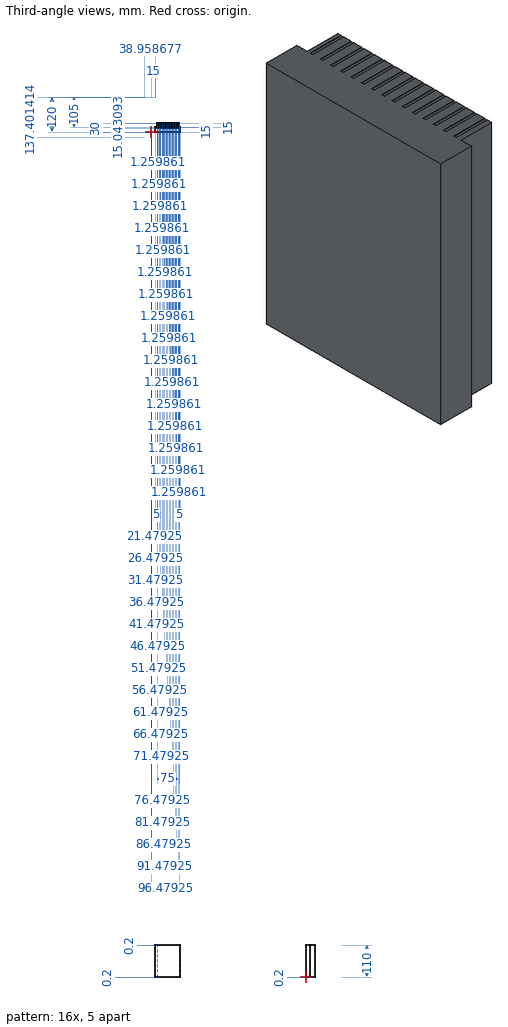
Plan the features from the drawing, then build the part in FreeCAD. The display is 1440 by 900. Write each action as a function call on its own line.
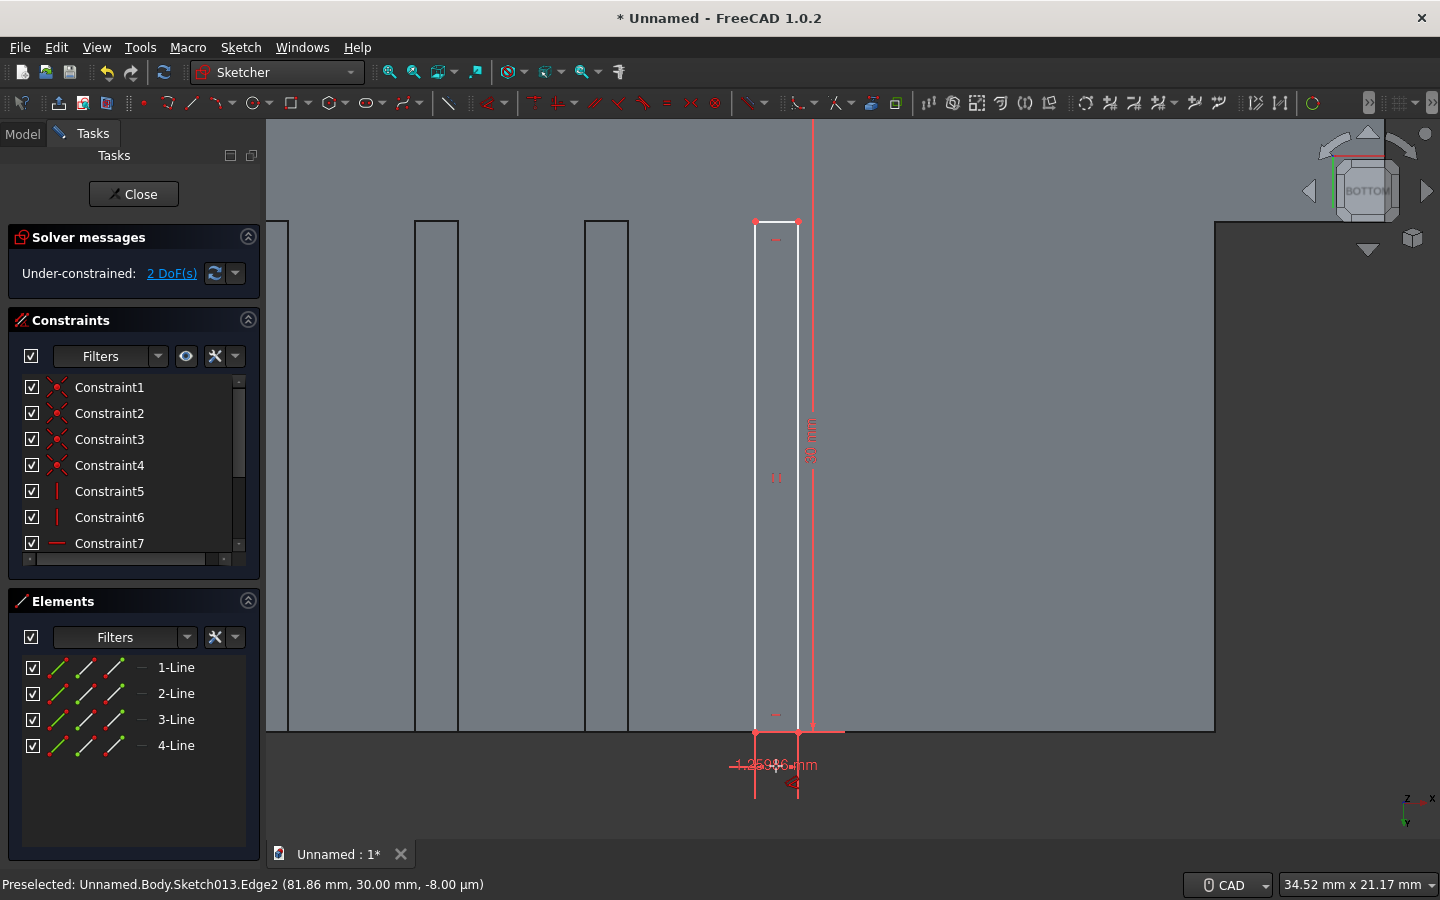
click(755, 375)
click(721, 477)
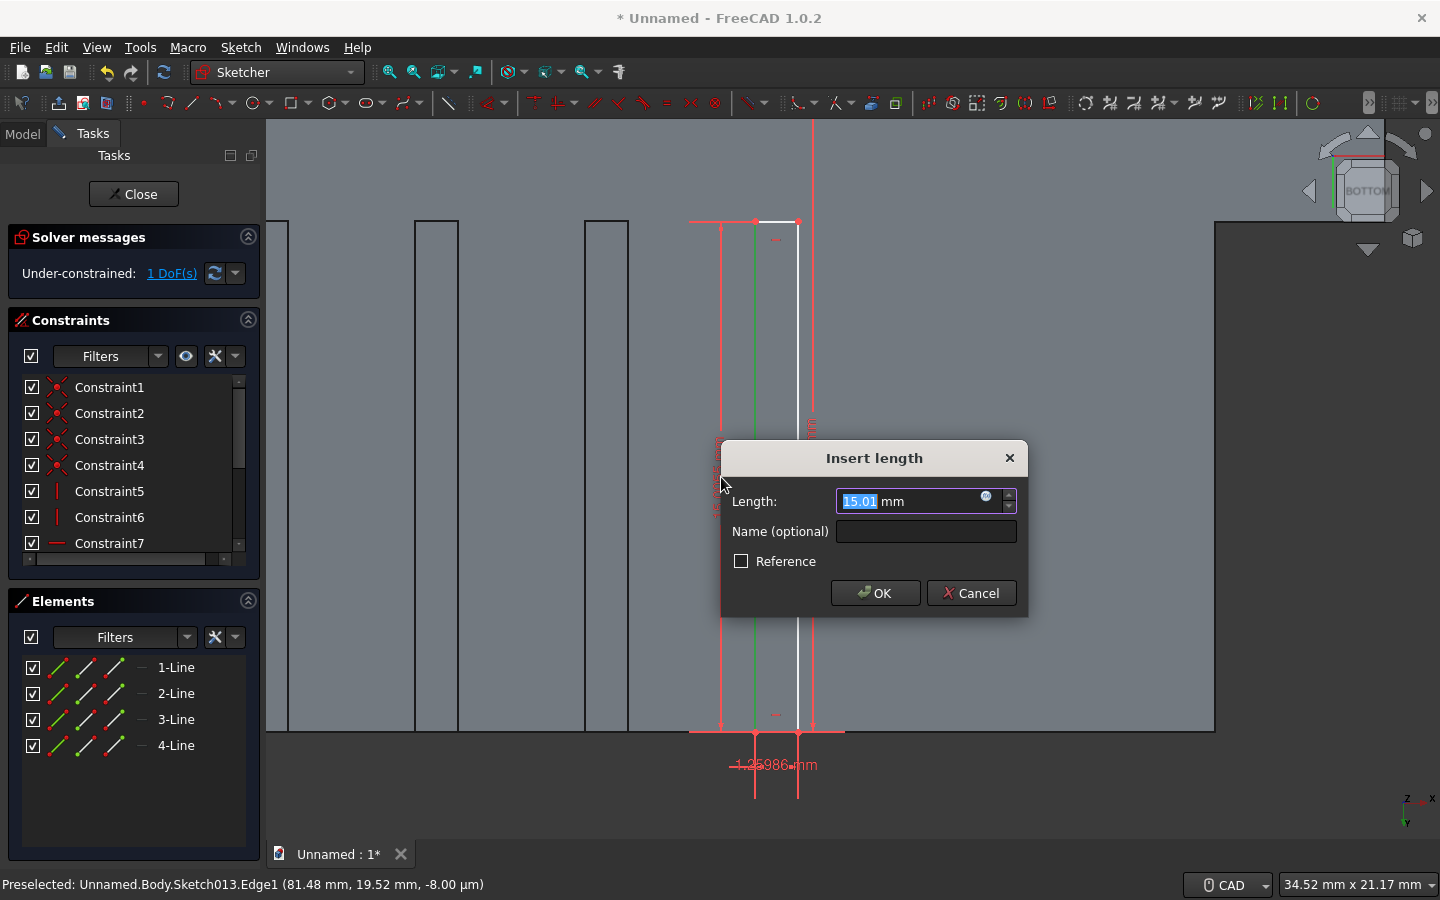
text(15.043093)
key(Return)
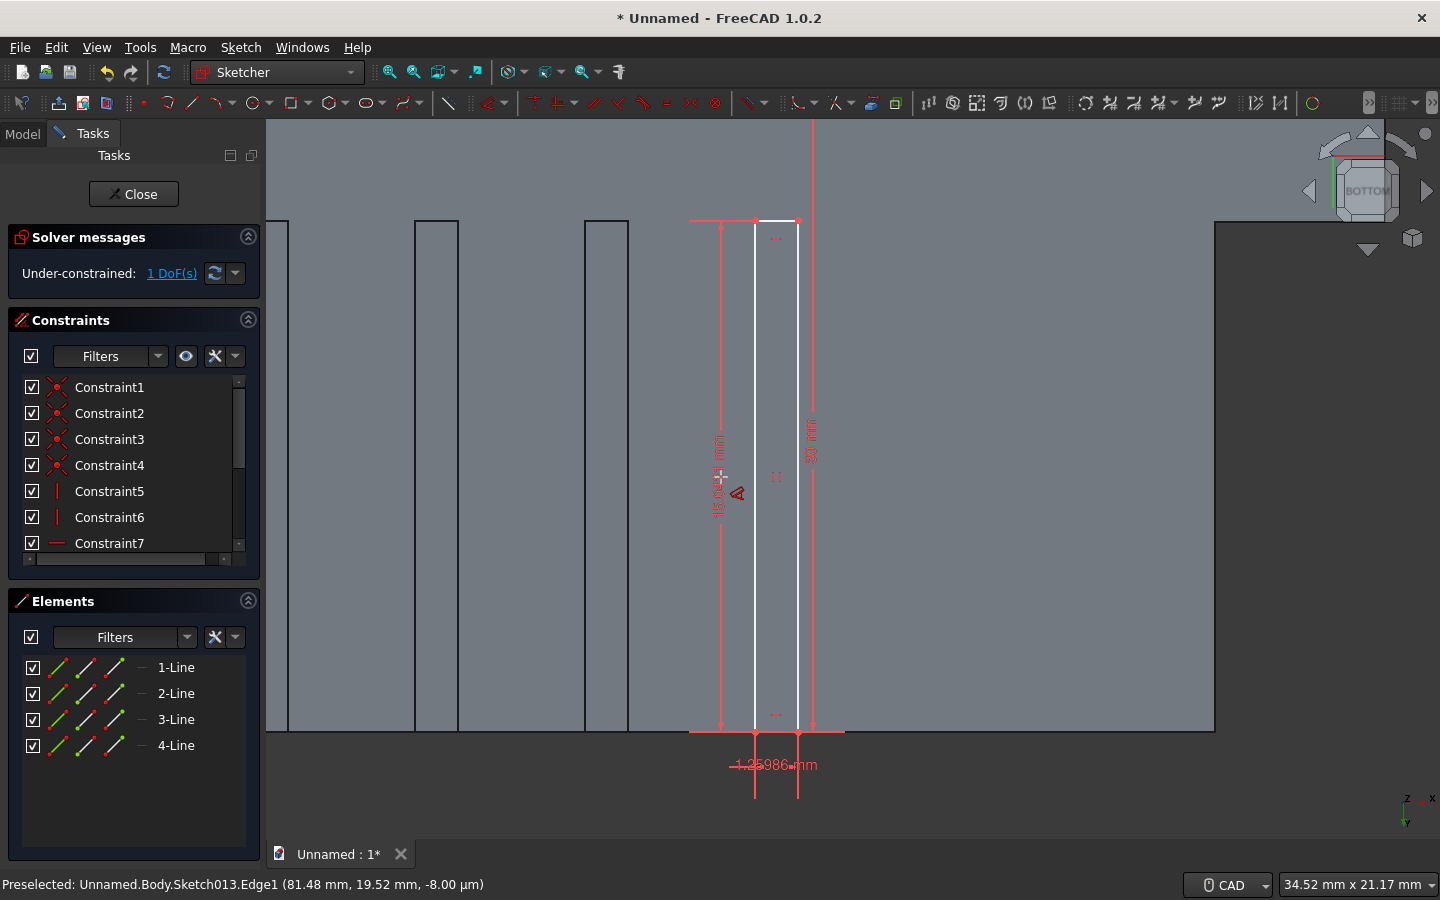
click(755, 221)
click(525, 255)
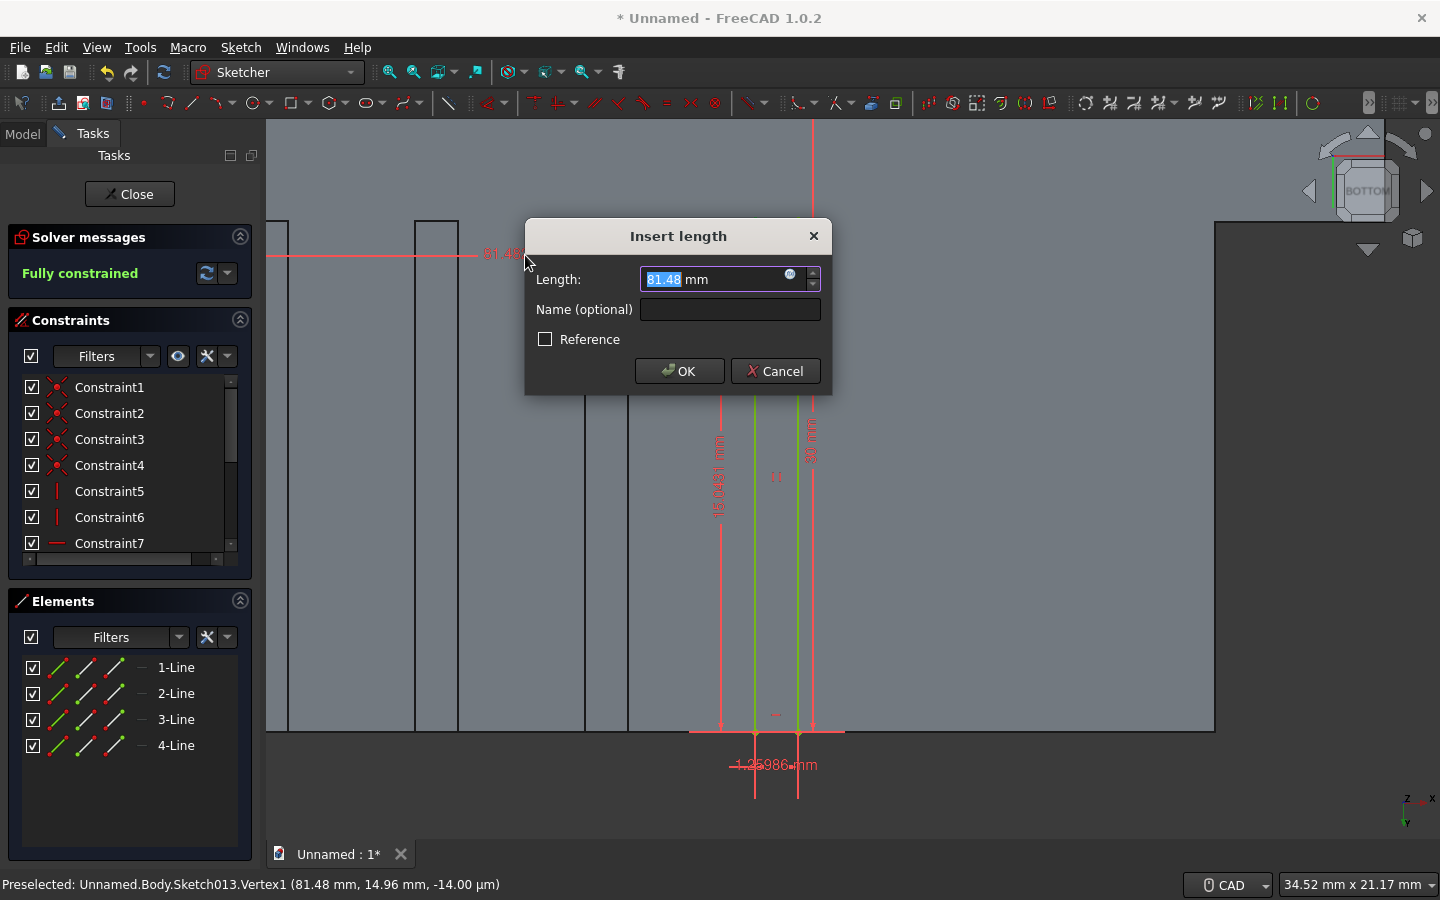
text(81.47925)
key(Return)
key(Escape)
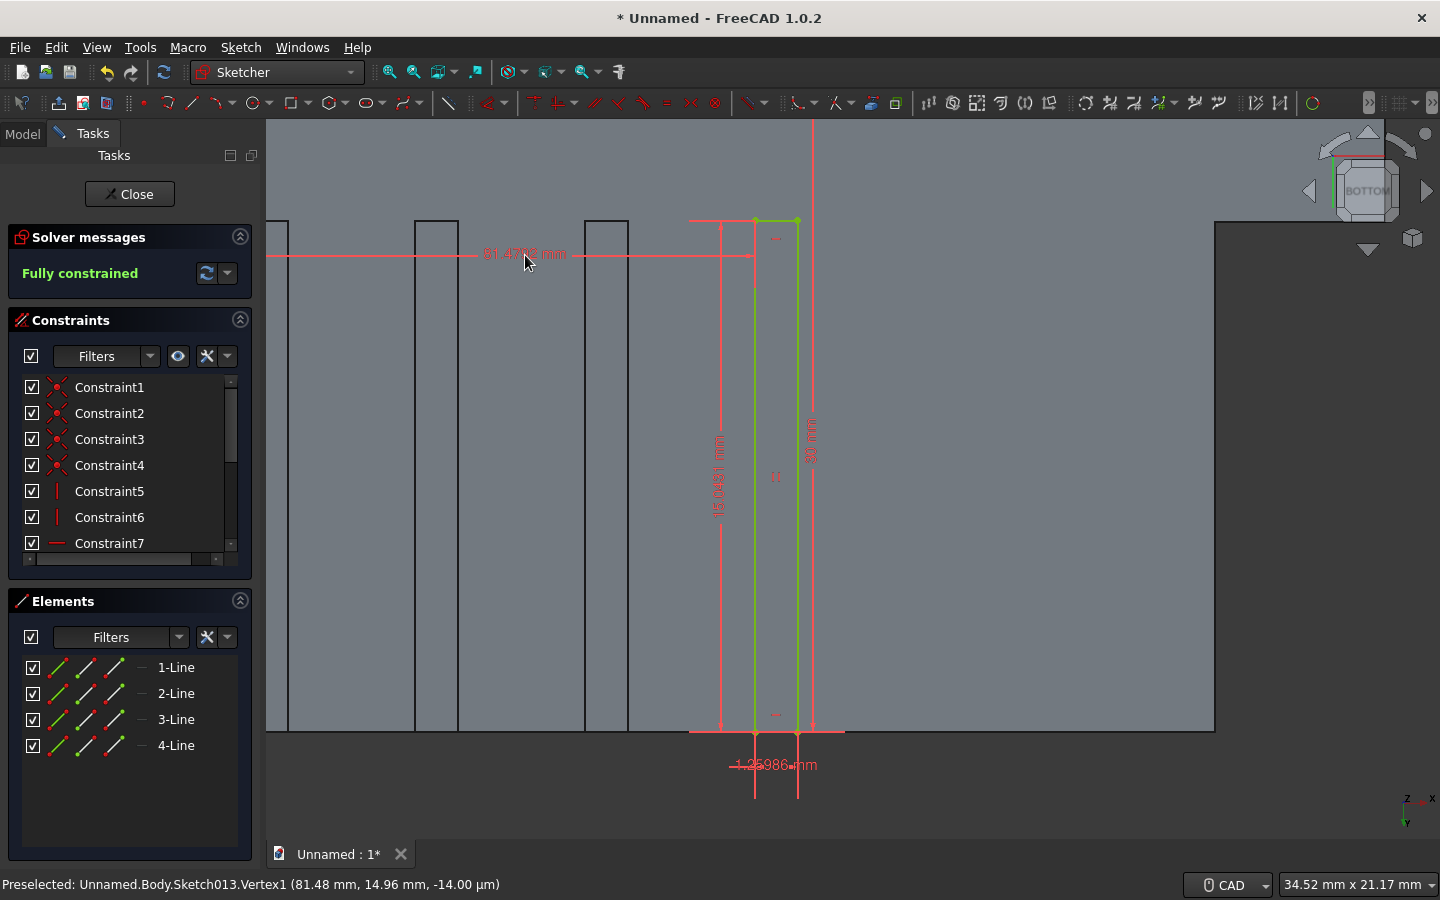
click(130, 194)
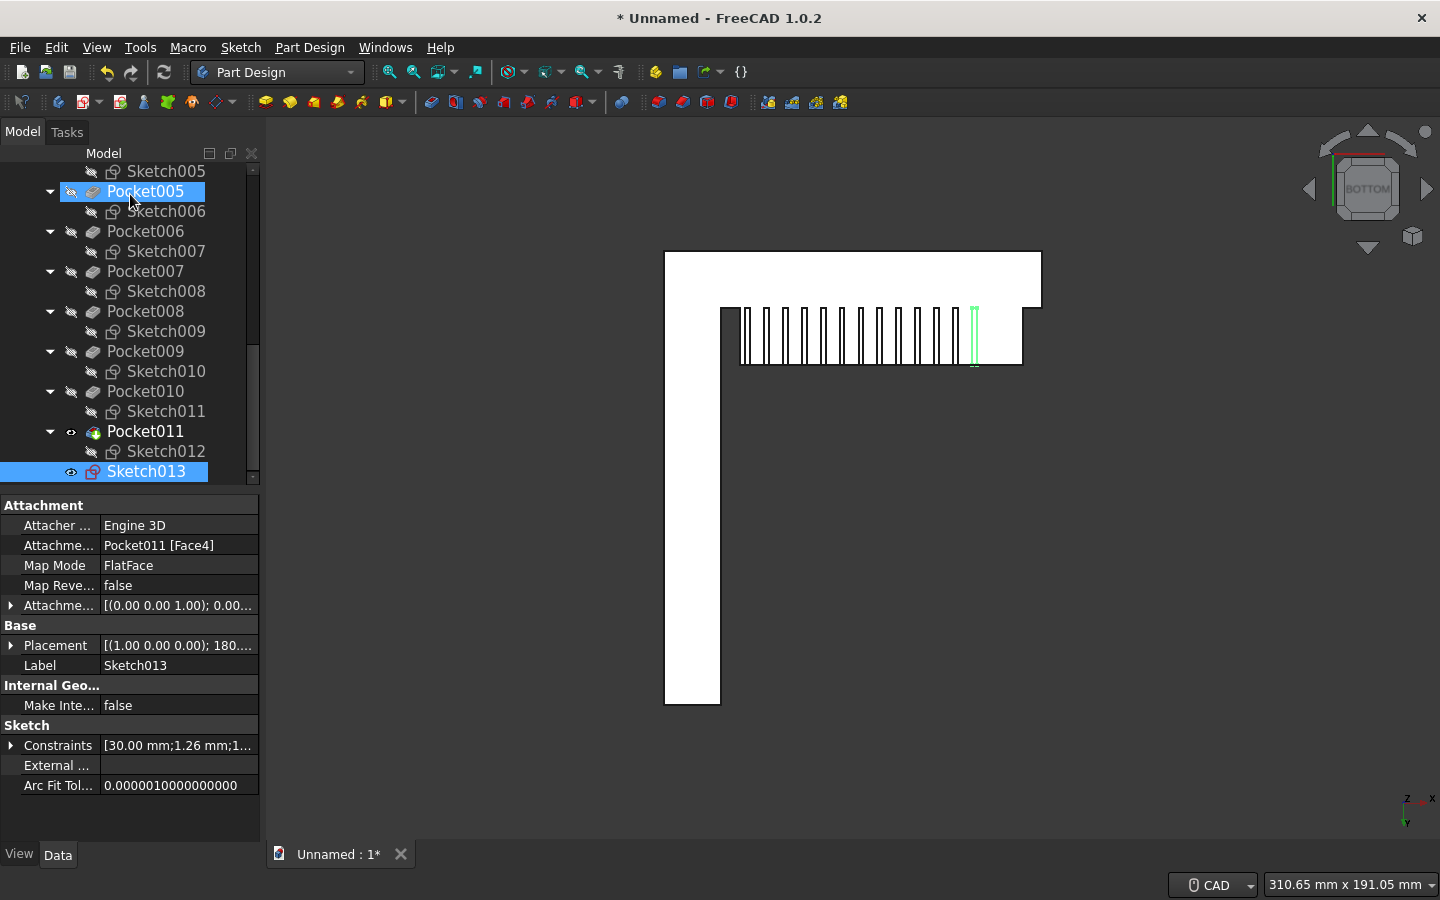
click(432, 102)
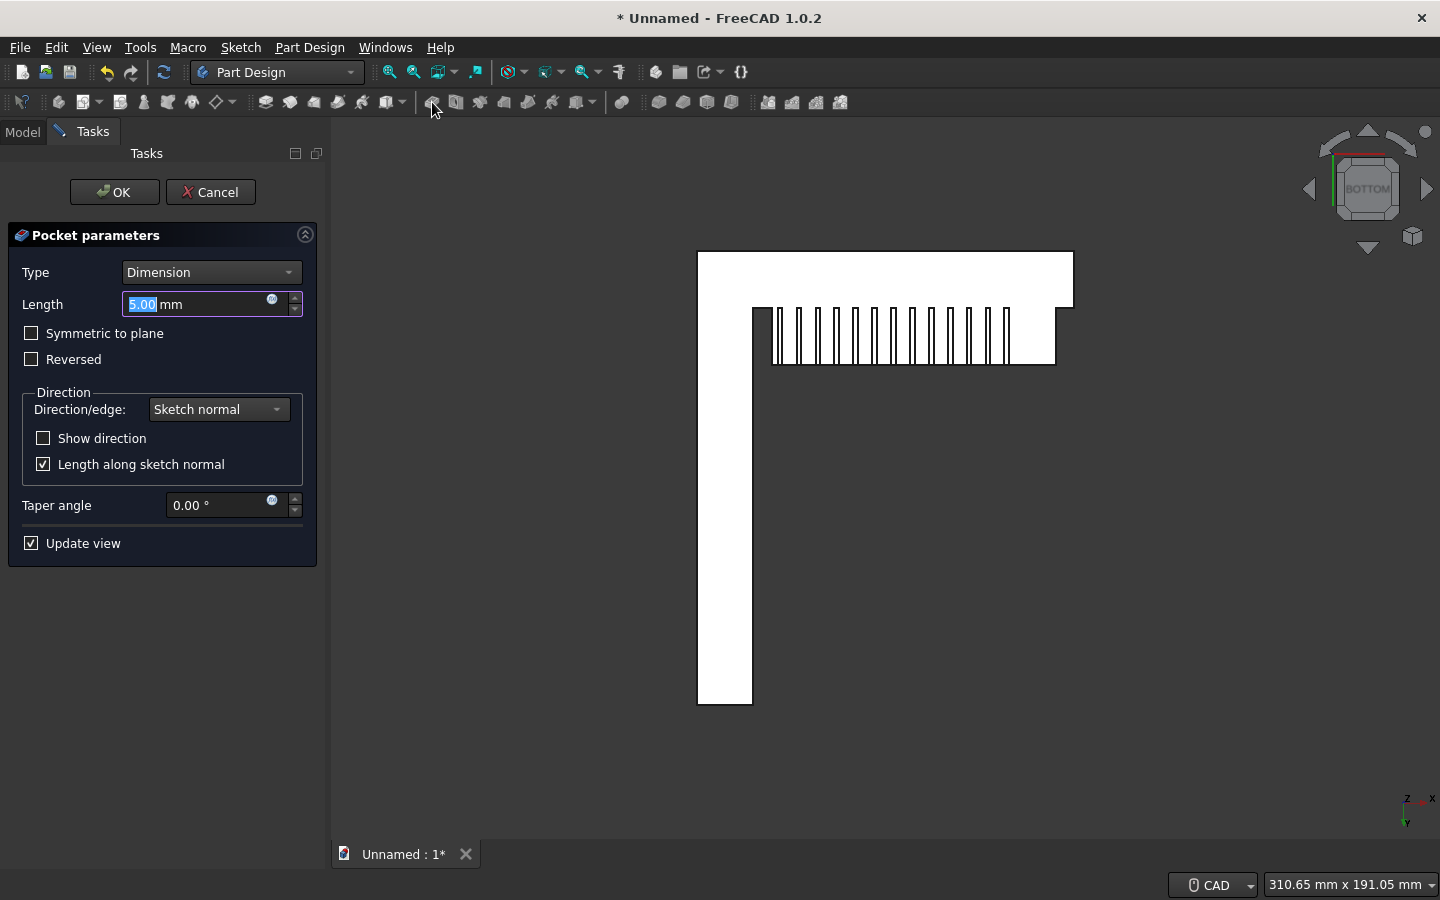
text(0.2)
key(Tab)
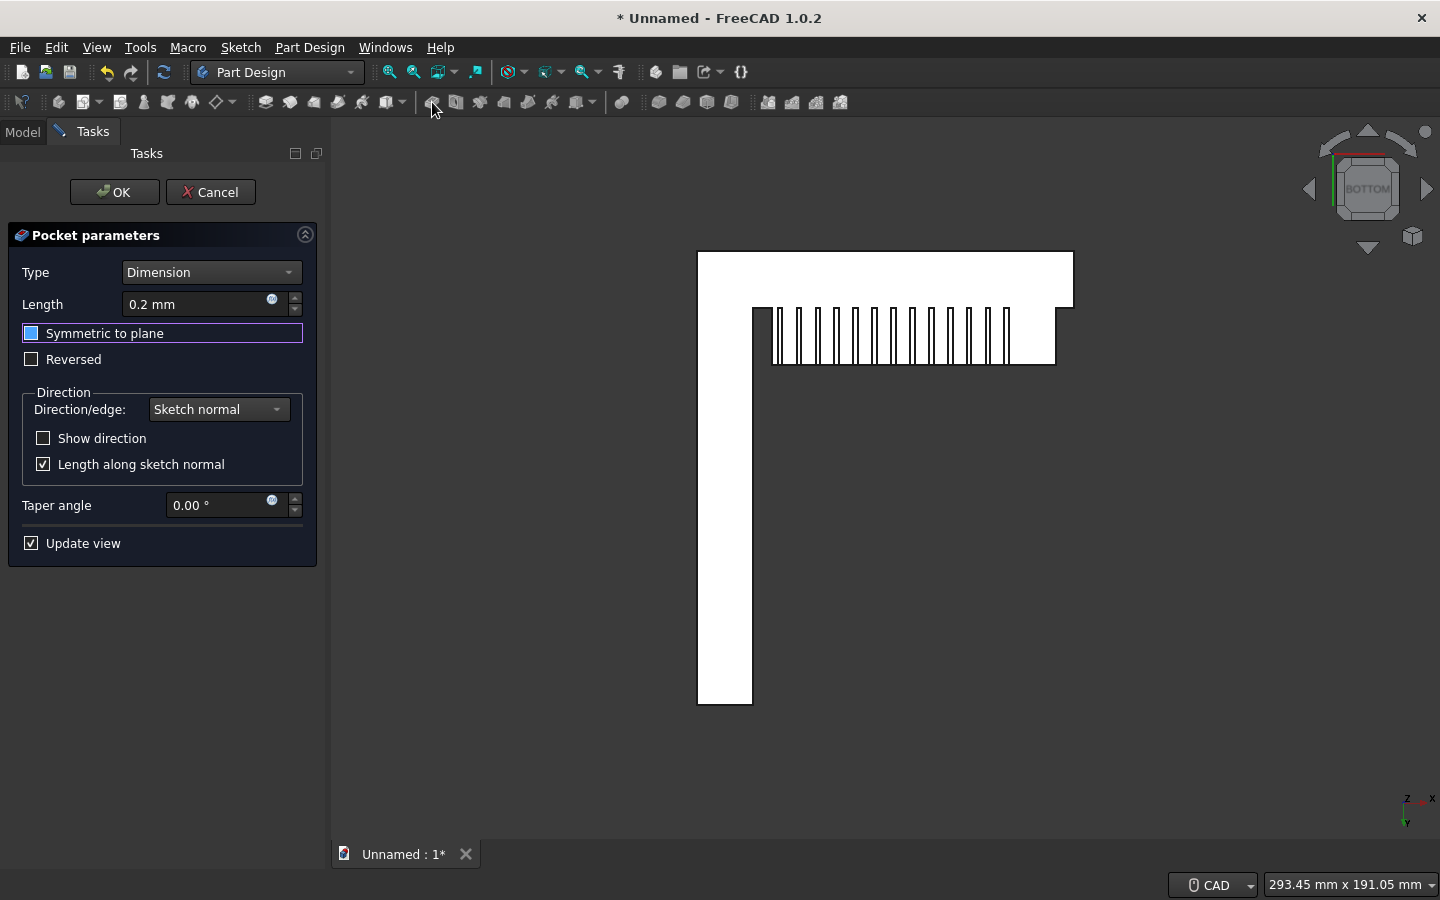
click(115, 192)